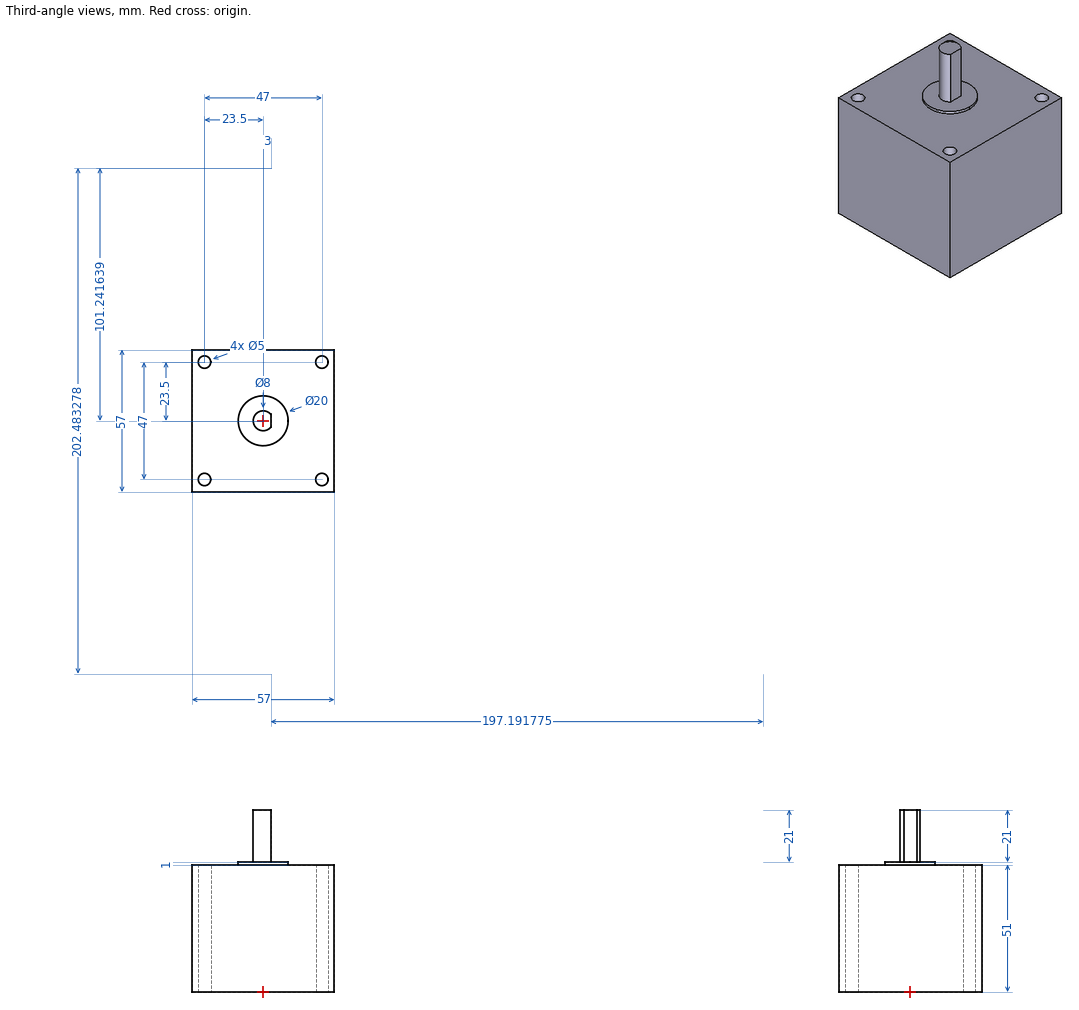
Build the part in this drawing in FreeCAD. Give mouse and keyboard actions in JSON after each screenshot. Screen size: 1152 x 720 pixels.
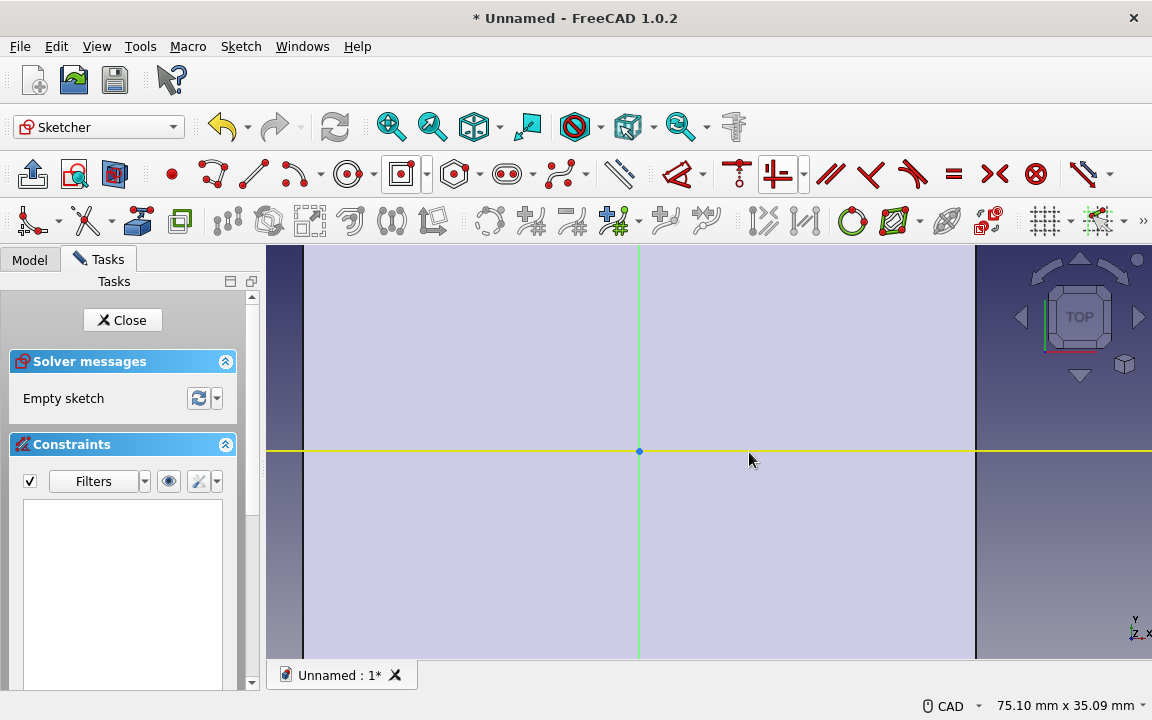
{"action": "left_click", "coordinate": [348, 174]}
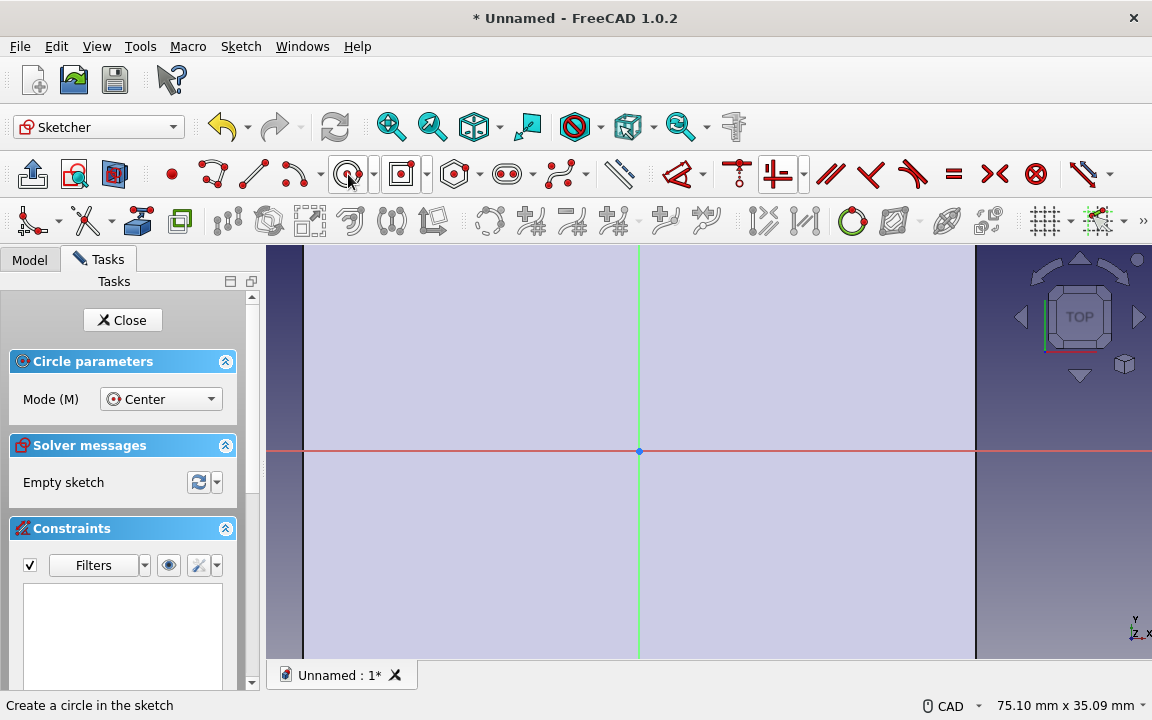
{"action": "left_click", "coordinate": [639, 451]}
{"action": "left_click", "coordinate": [723, 368]}
{"action": "key", "text": "Escape"}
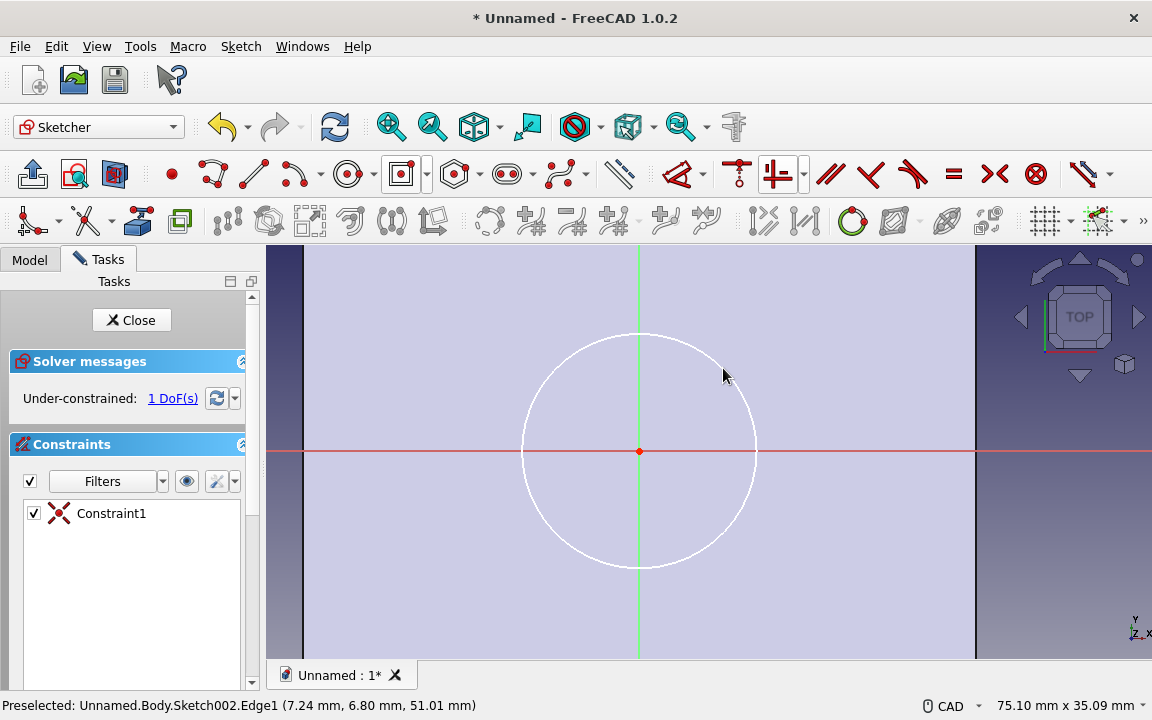
{"action": "left_click", "coordinate": [676, 174]}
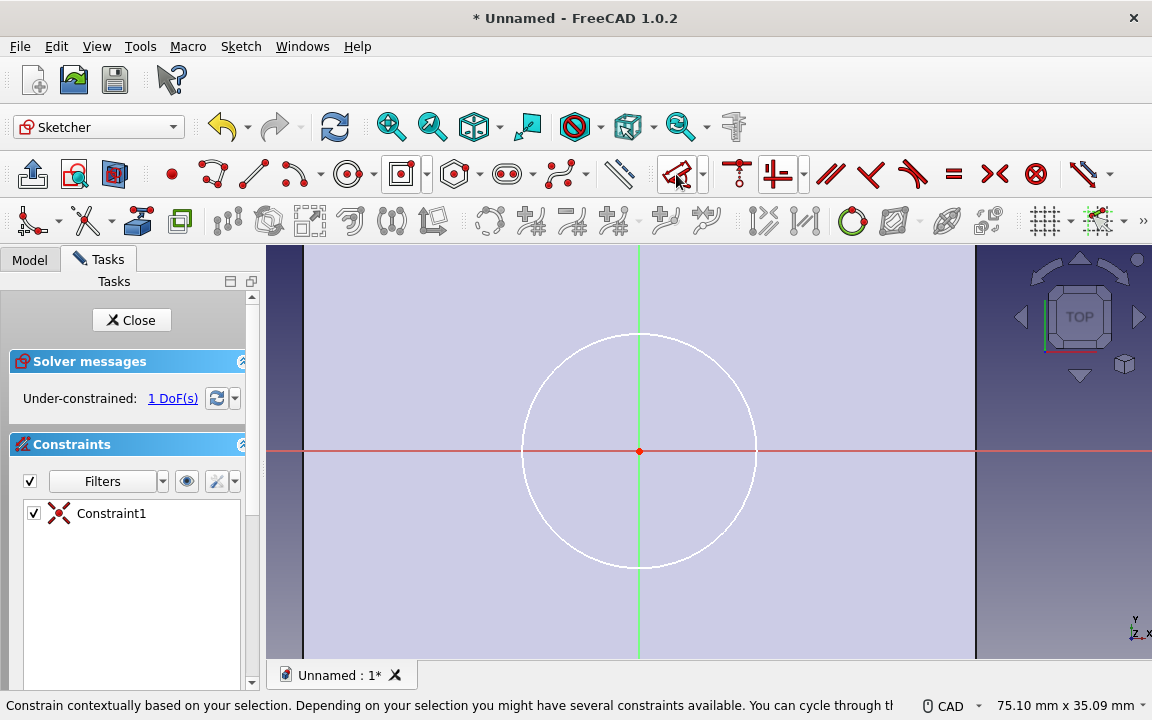
{"action": "left_click", "coordinate": [722, 368]}
{"action": "left_click", "coordinate": [745, 345]}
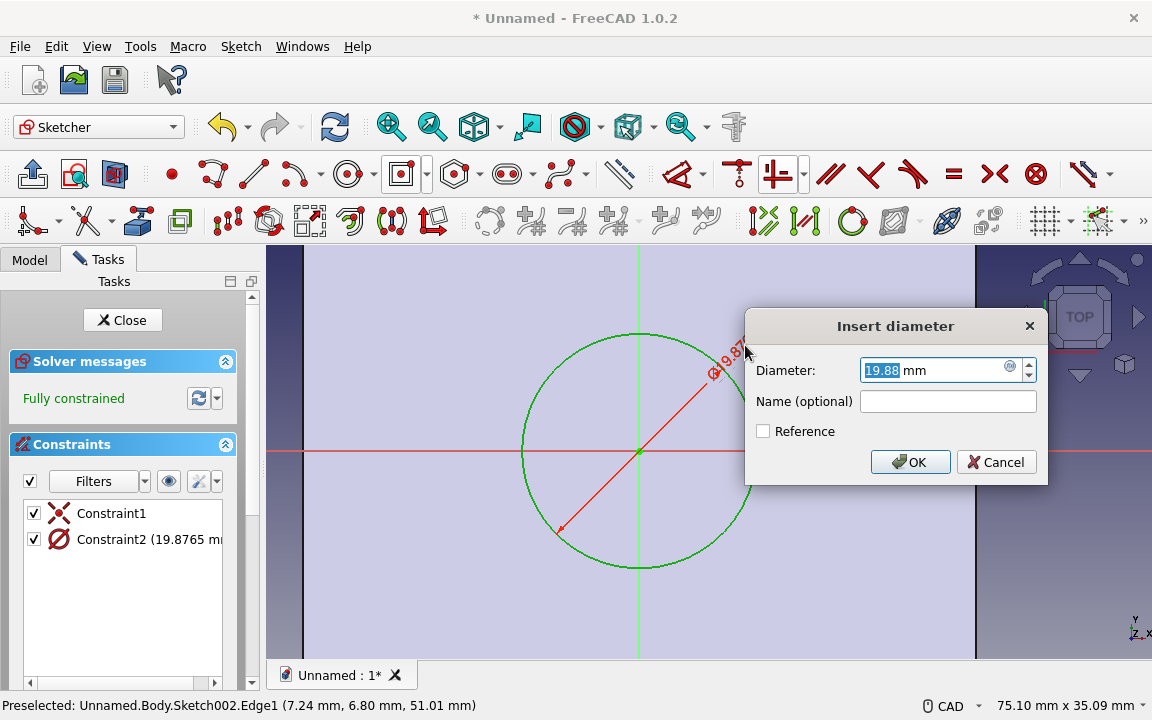
{"action": "type", "text": "20"}
{"action": "key", "text": "Return"}
{"action": "key", "text": "Escape"}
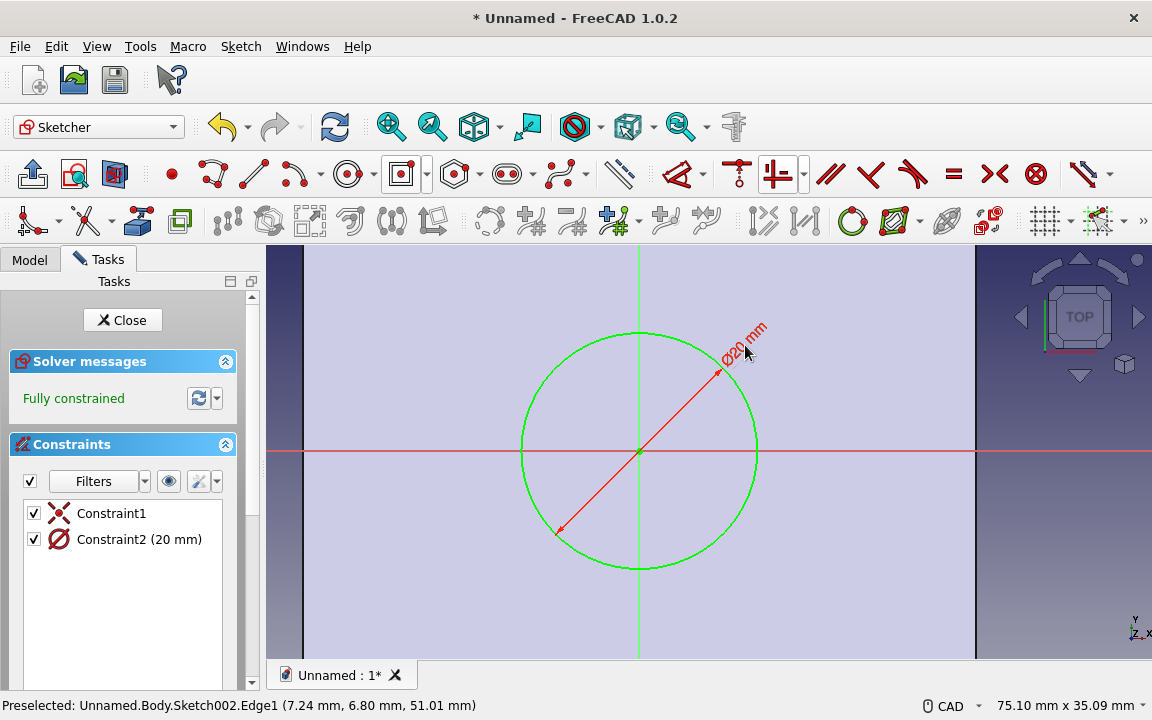
{"action": "left_click", "coordinate": [123, 320]}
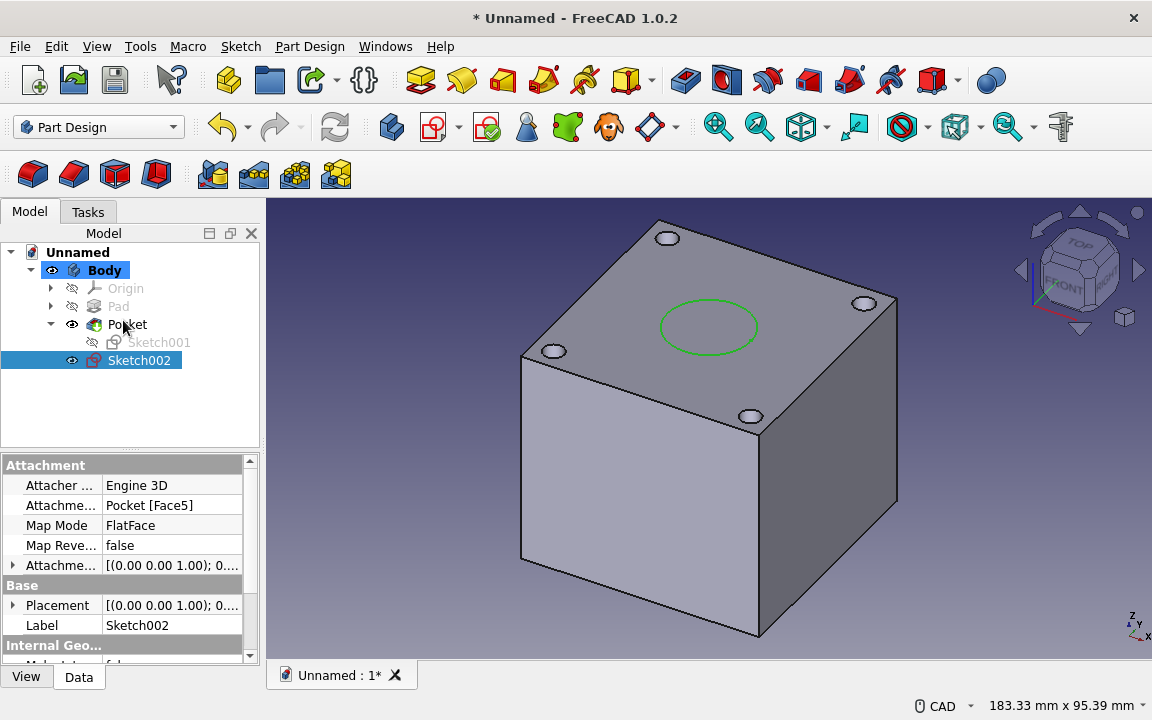
{"action": "left_click", "coordinate": [421, 80]}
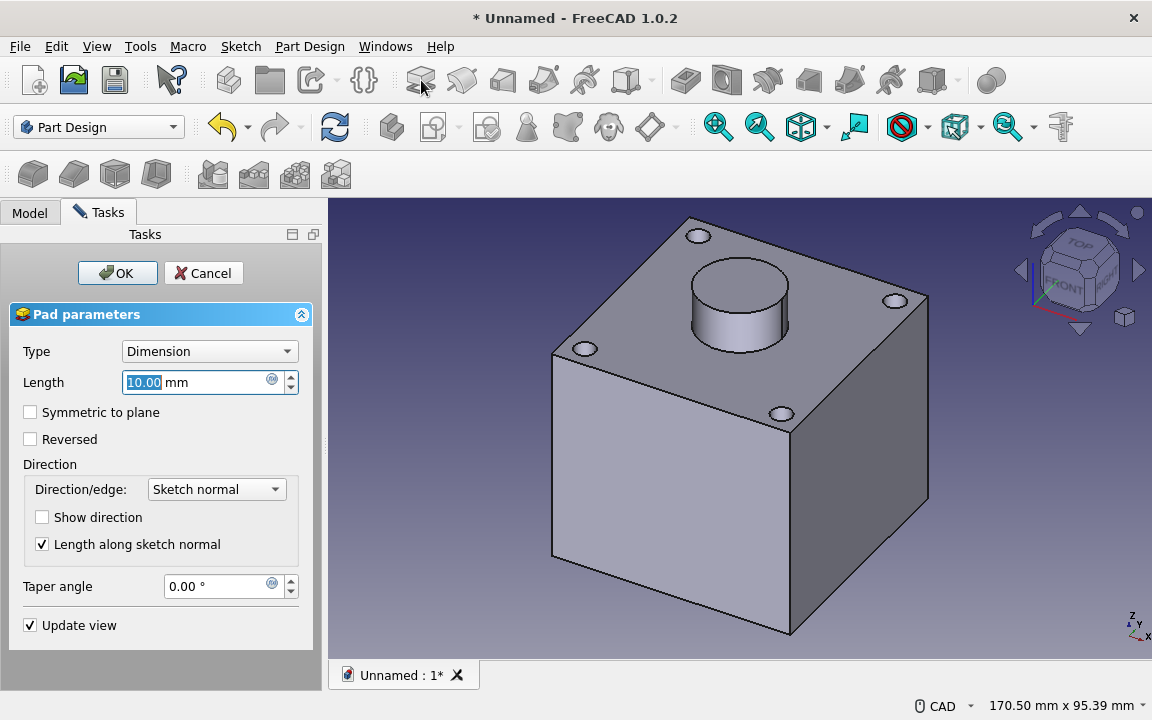
{"action": "type", "text": "1"}
{"action": "key", "text": "Tab"}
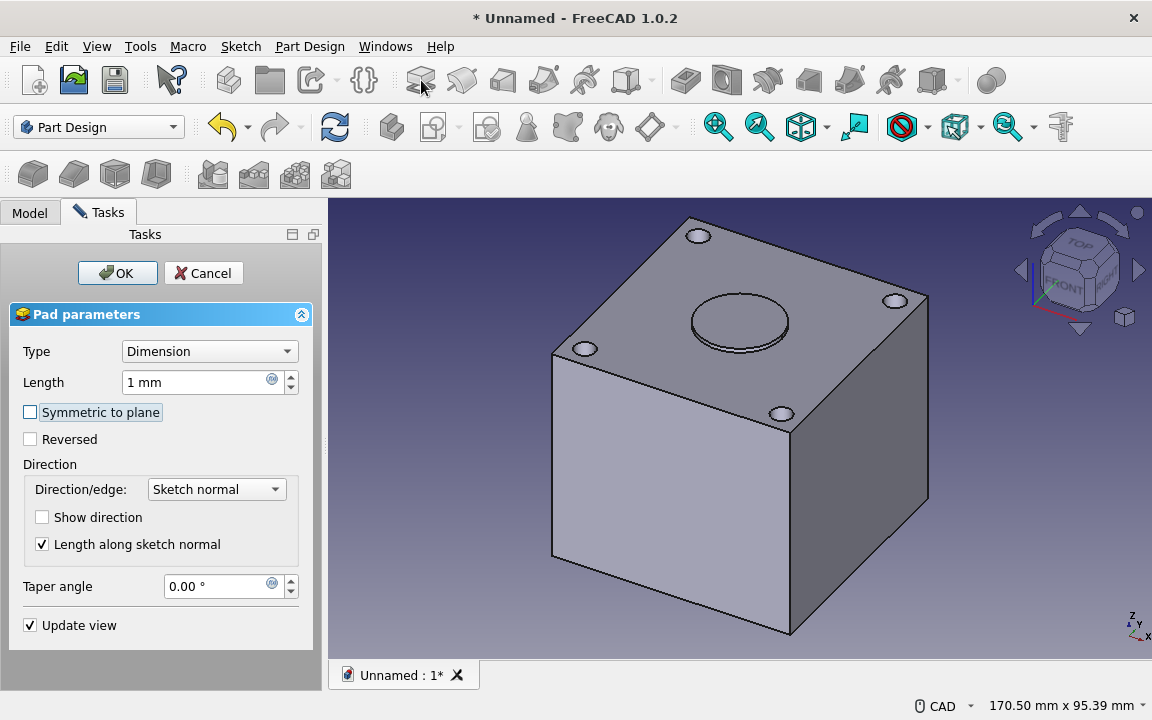
{"action": "left_click", "coordinate": [118, 273]}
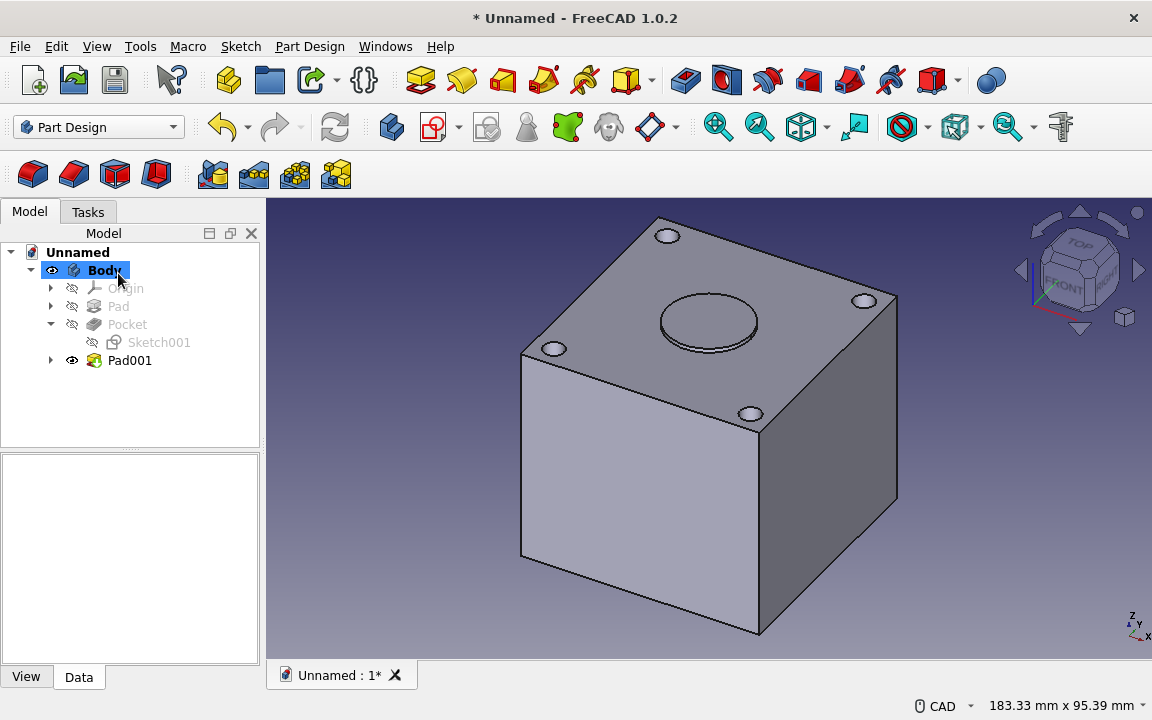
{"action": "left_click", "coordinate": [709, 320]}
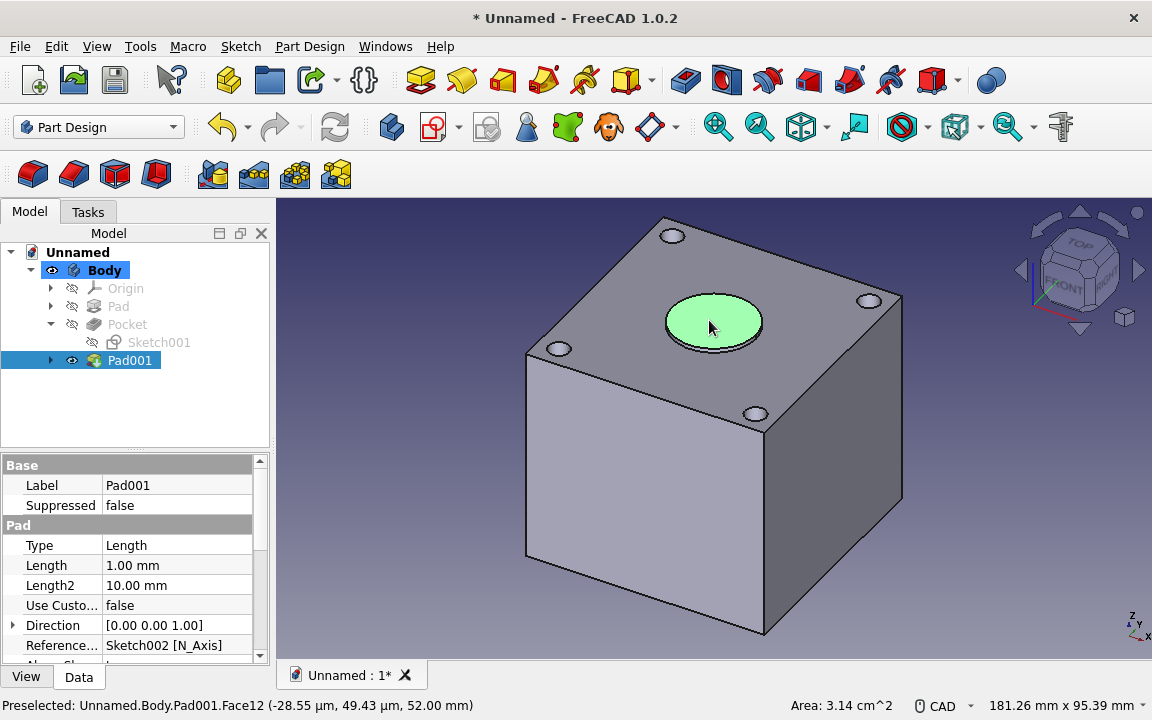
{"action": "left_click", "coordinate": [432, 128]}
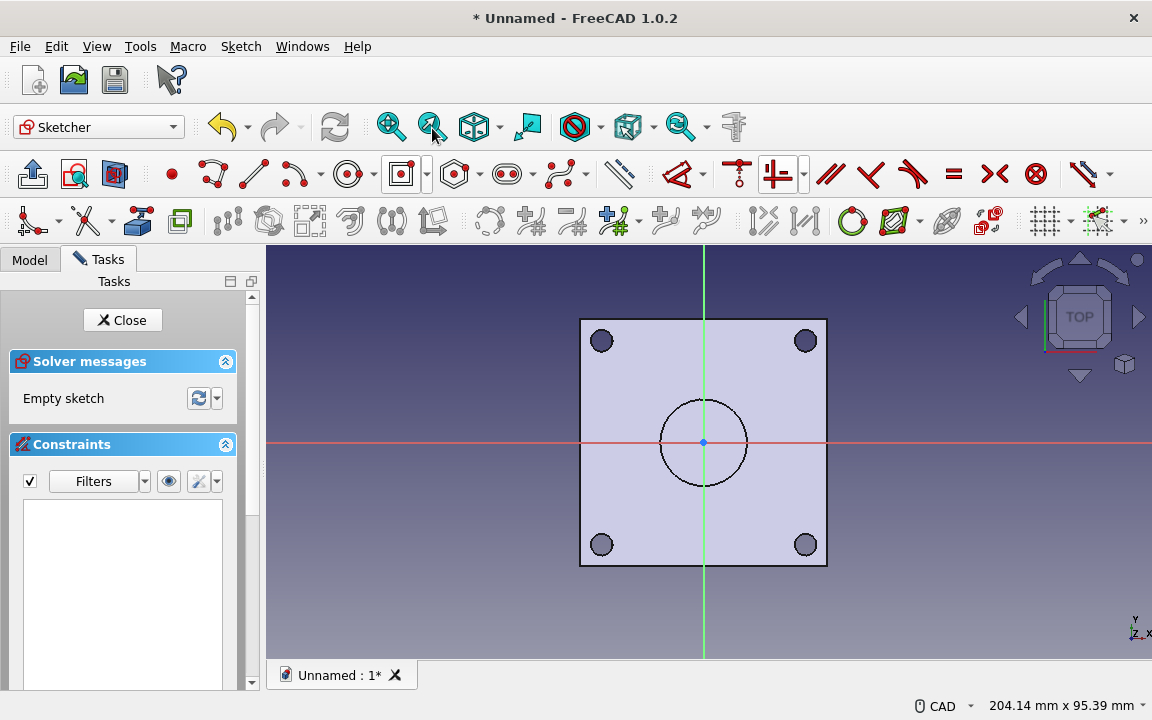
{"action": "scroll", "coordinate": [714, 441], "scroll_direction": "up", "scroll_amount": 10}